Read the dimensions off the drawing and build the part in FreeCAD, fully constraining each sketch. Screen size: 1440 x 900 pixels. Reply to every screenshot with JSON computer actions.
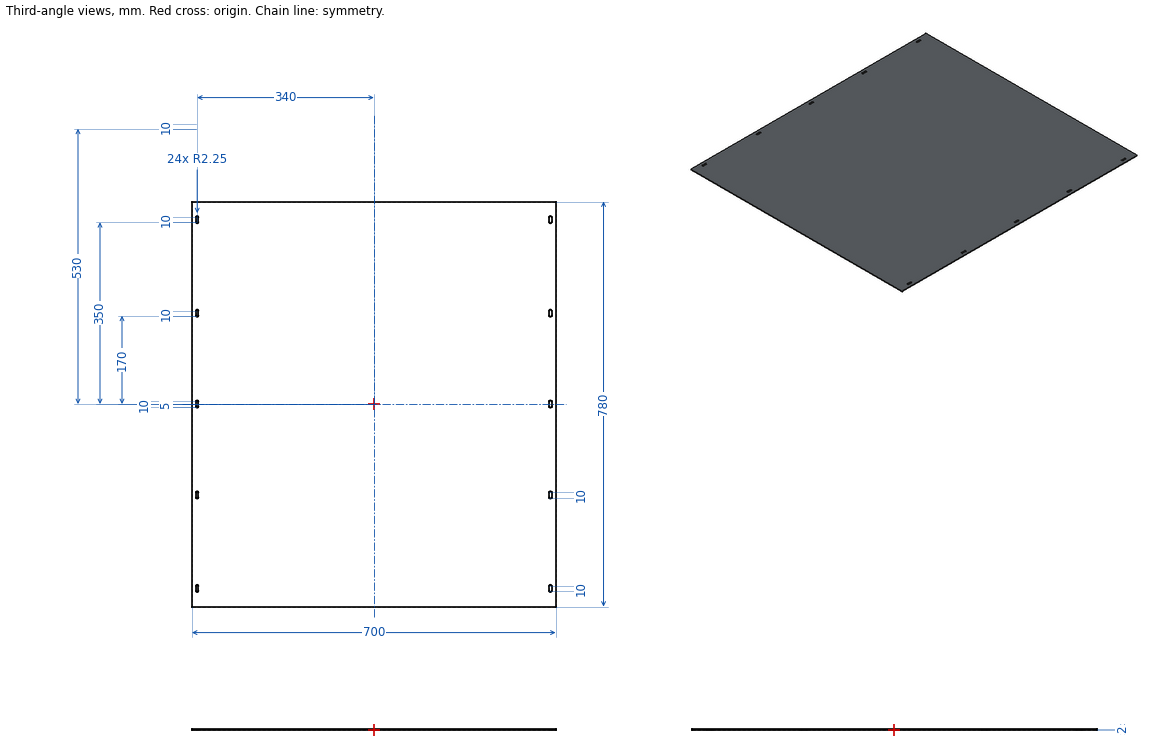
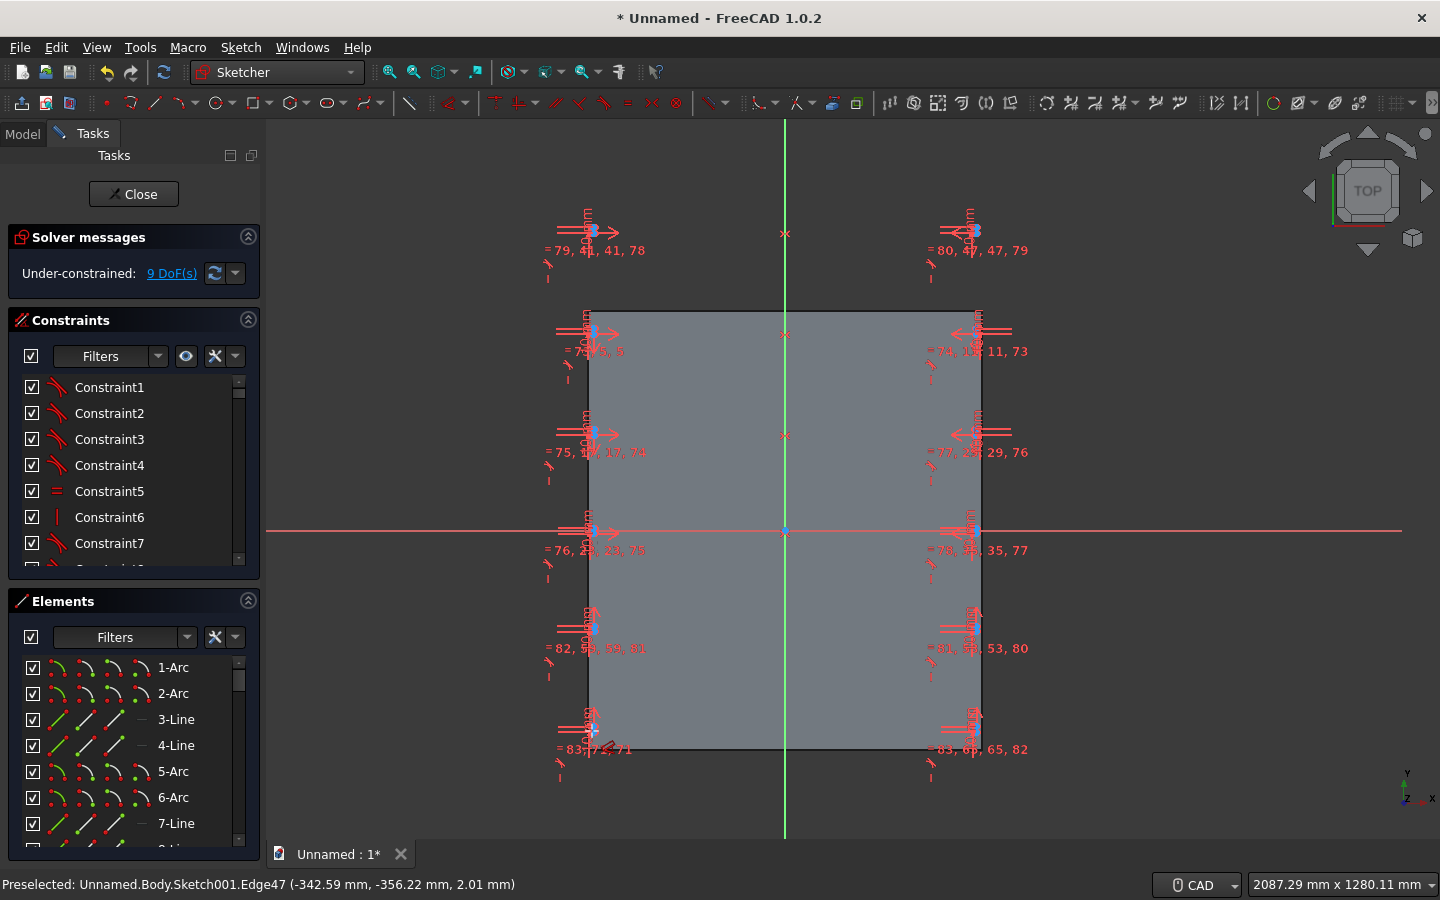
{"action": "scroll", "coordinate": [593, 534], "scroll_direction": "up", "scroll_amount": 14}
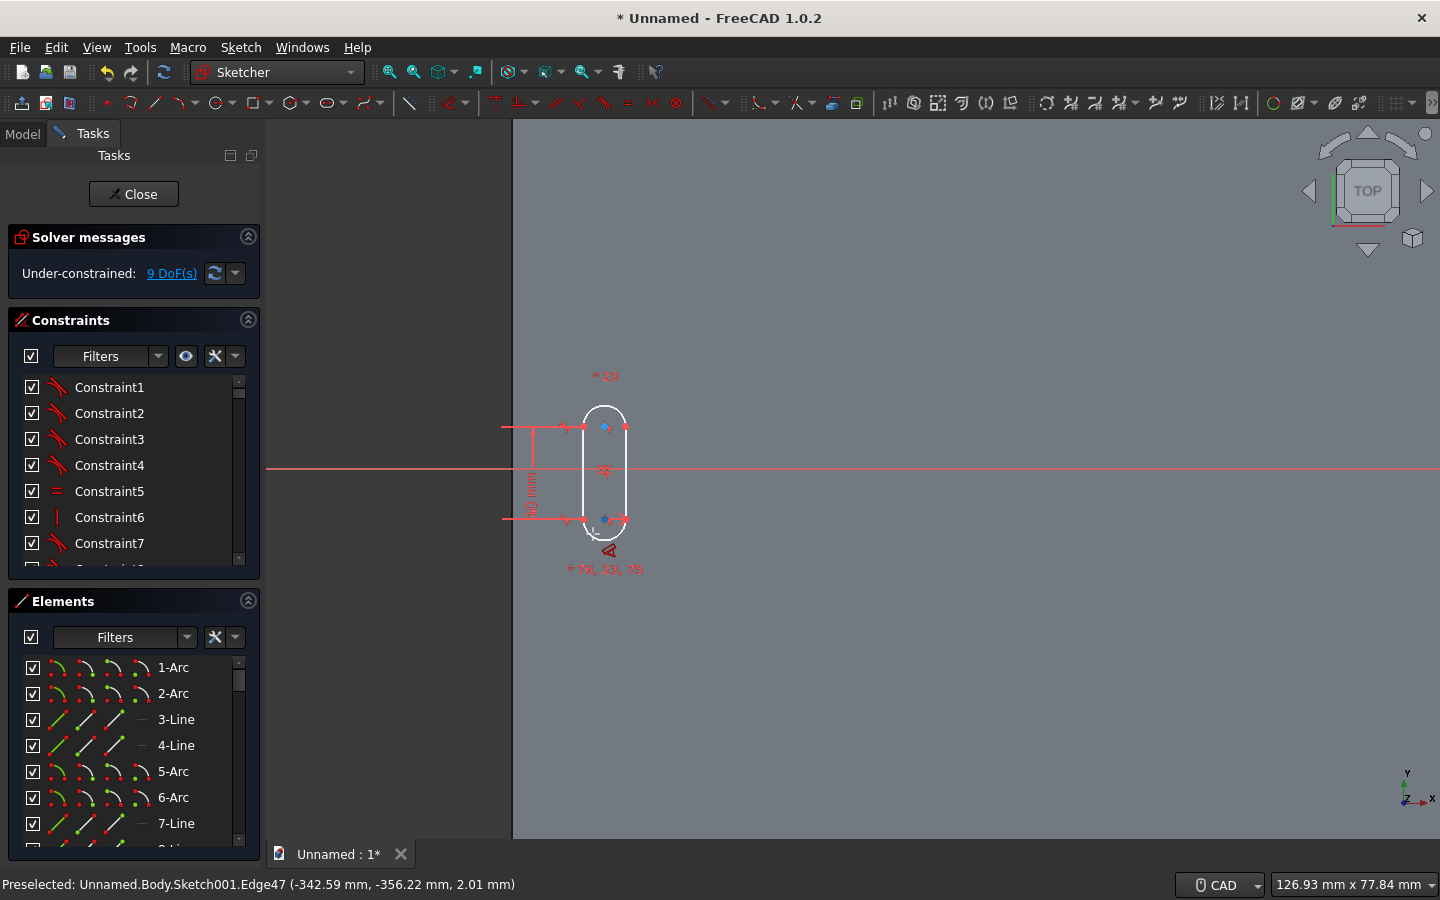
{"action": "left_click", "coordinate": [583, 519]}
{"action": "left_click", "coordinate": [453, 494]}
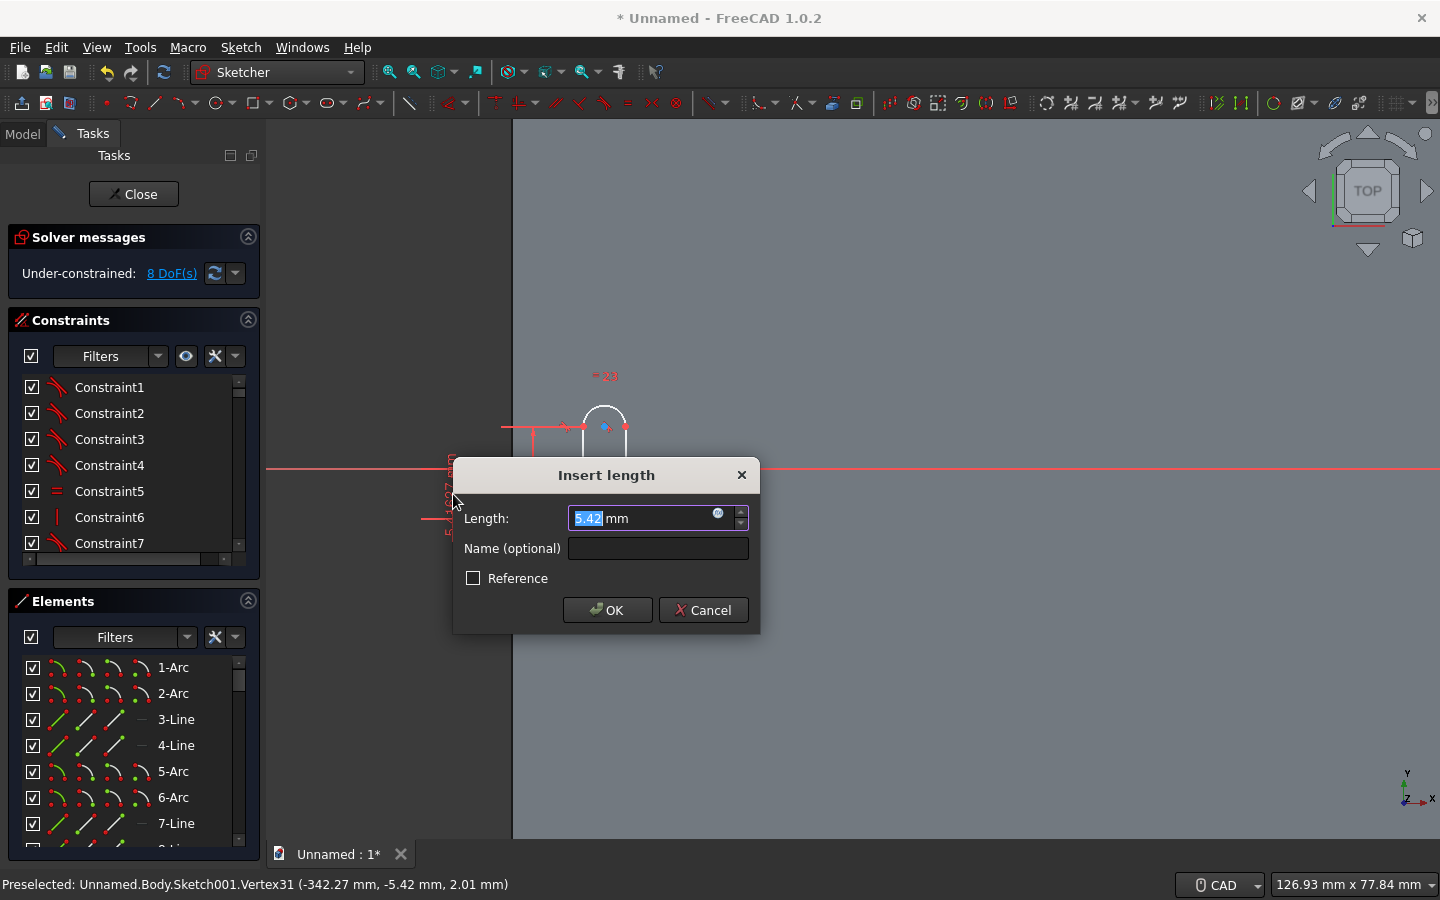
{"action": "type", "text": "5"}
{"action": "key", "text": "Return"}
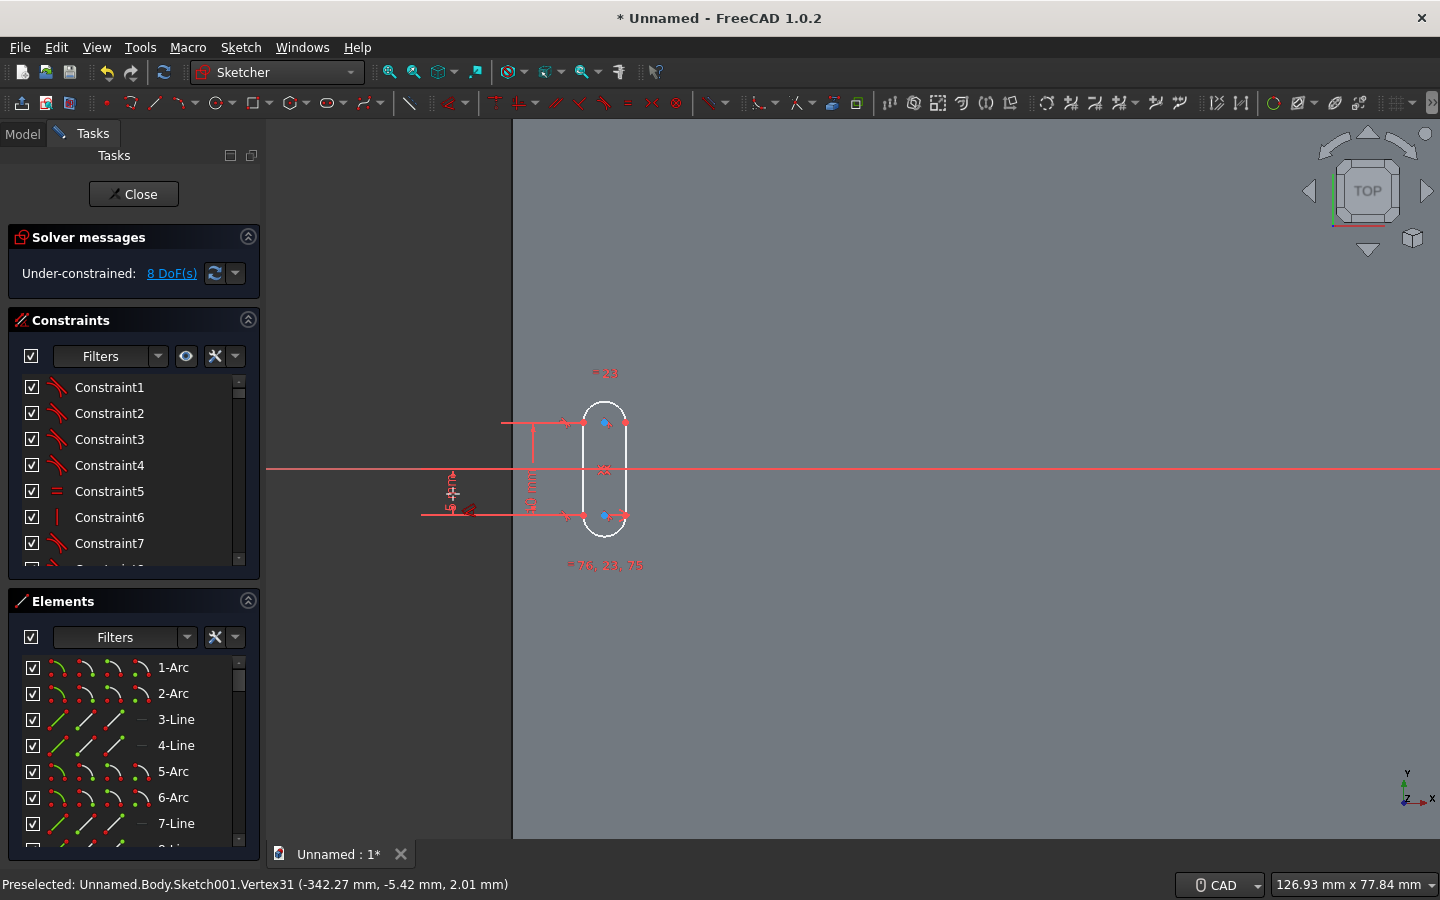
{"action": "scroll", "coordinate": [593, 534], "scroll_direction": "down", "scroll_amount": 14}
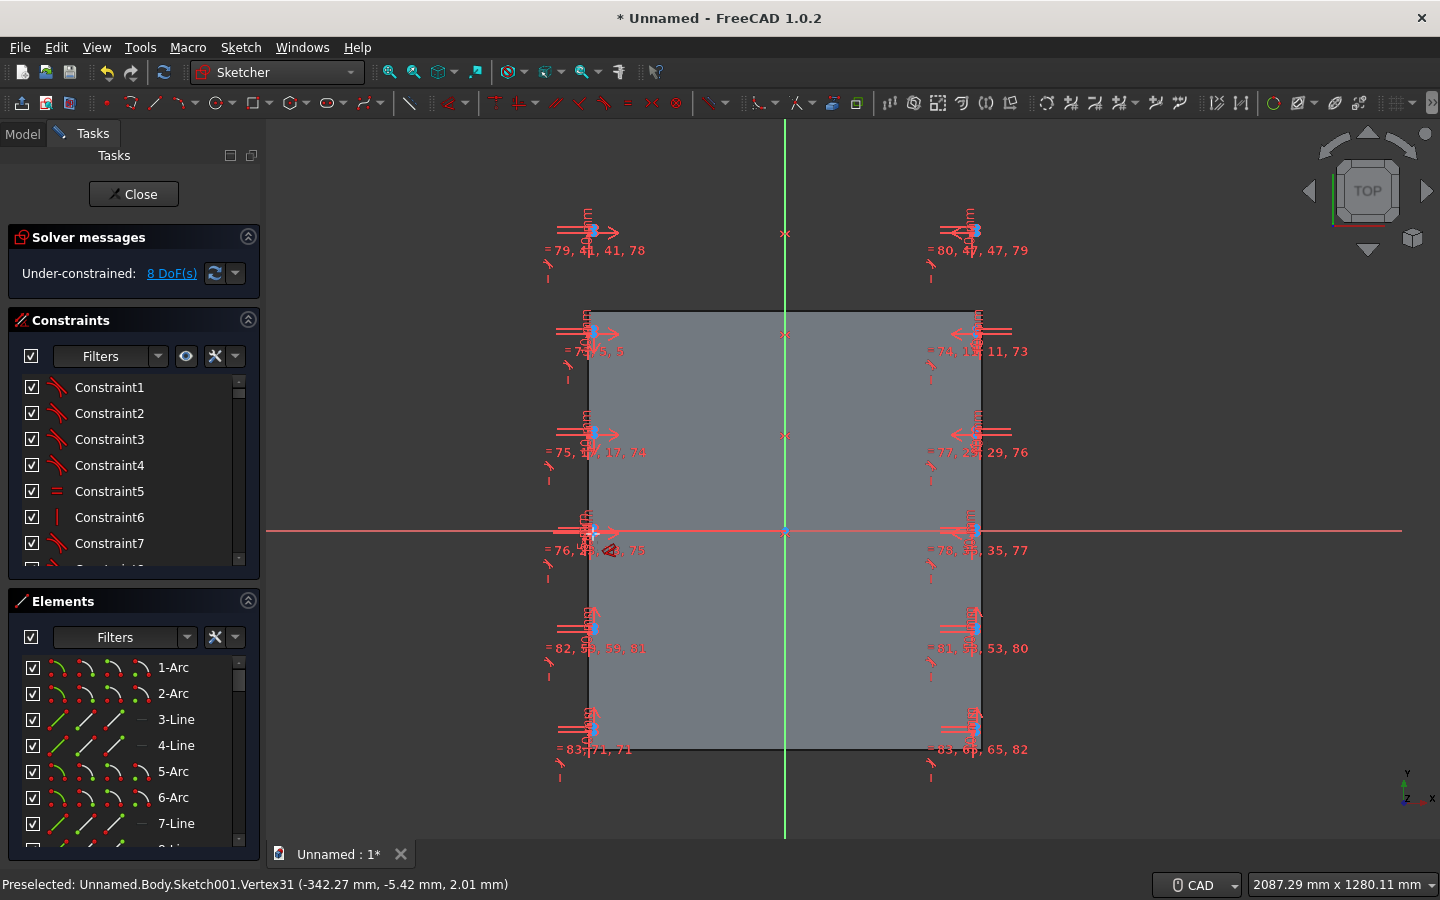
{"action": "scroll", "coordinate": [593, 334], "scroll_direction": "up", "scroll_amount": 12}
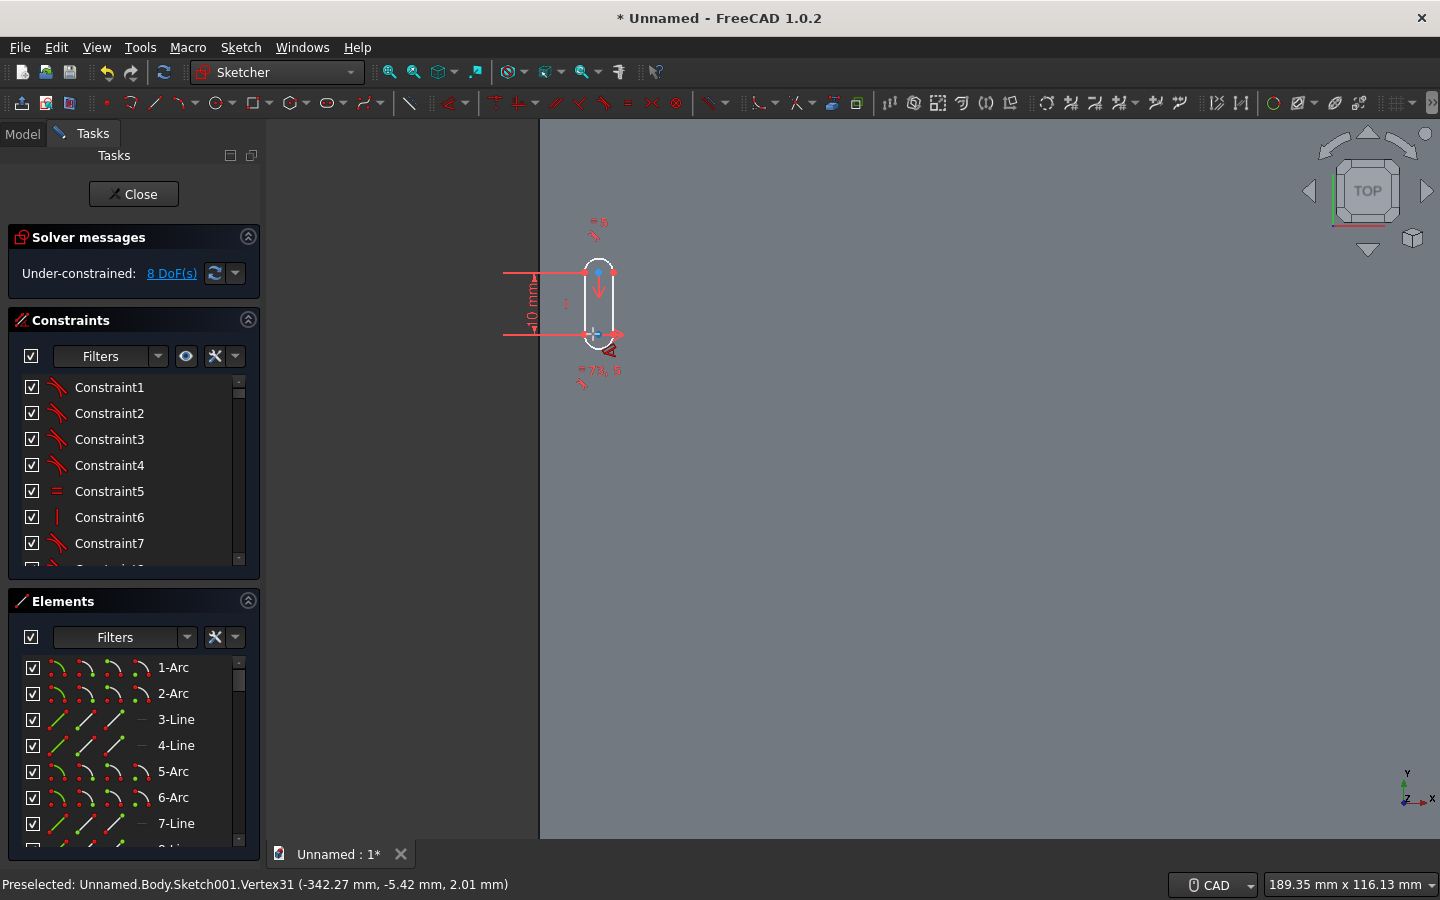
{"action": "left_click", "coordinate": [585, 335]}
{"action": "left_click", "coordinate": [551, 573]}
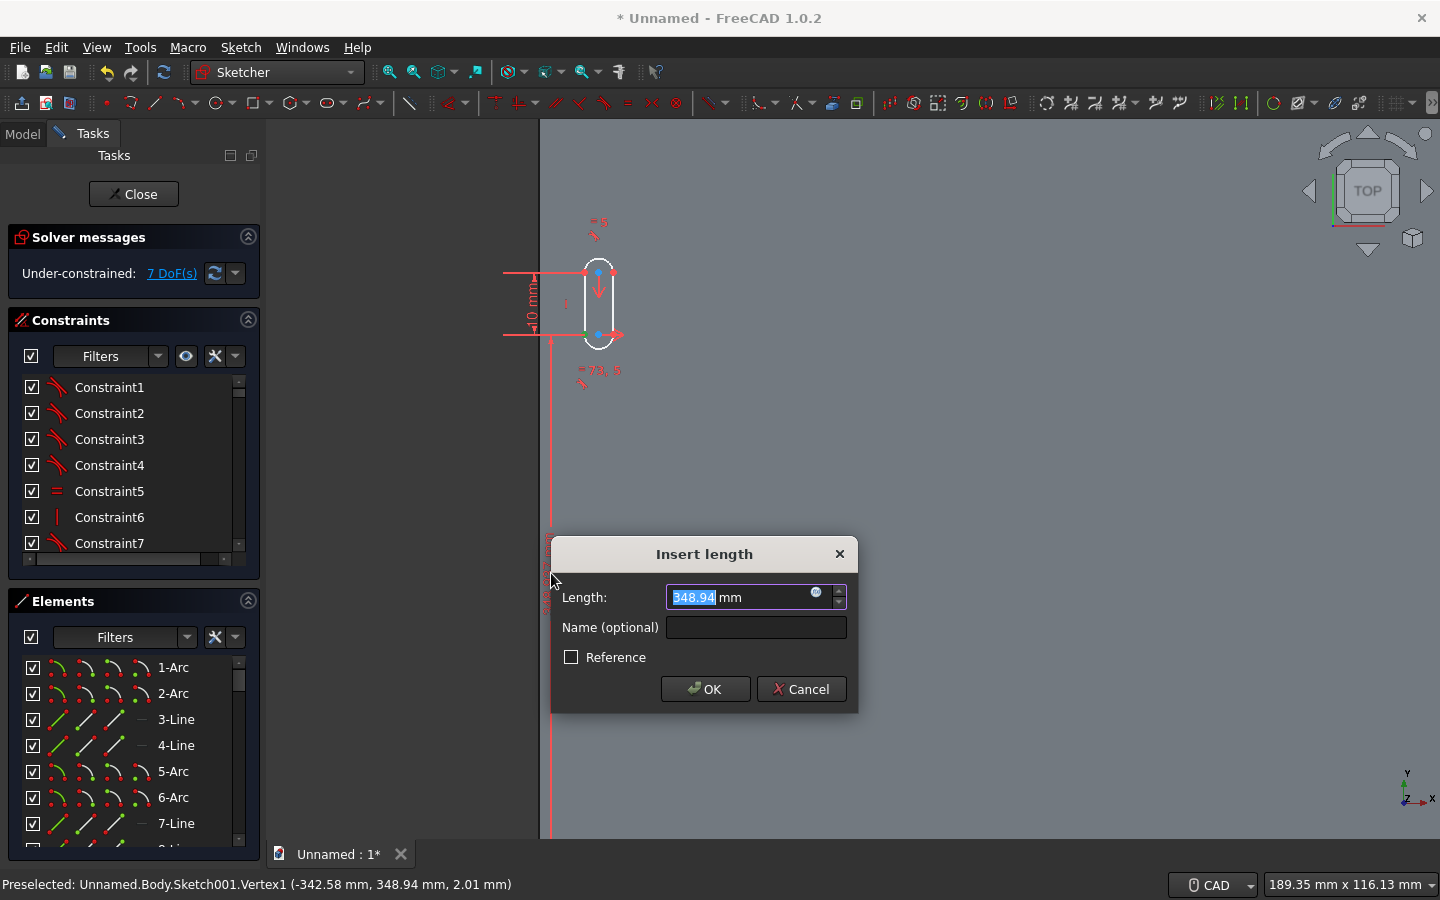
{"action": "type", "text": "350"}
{"action": "key", "text": "Return"}